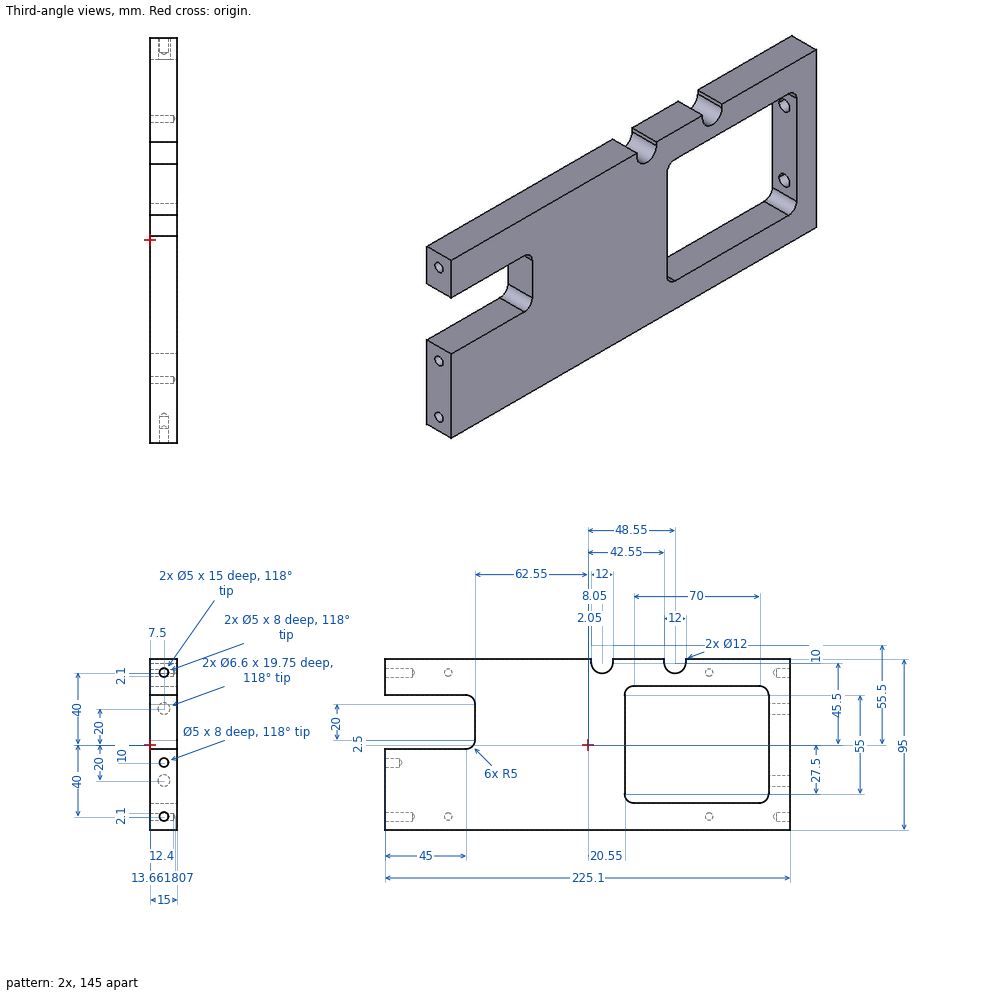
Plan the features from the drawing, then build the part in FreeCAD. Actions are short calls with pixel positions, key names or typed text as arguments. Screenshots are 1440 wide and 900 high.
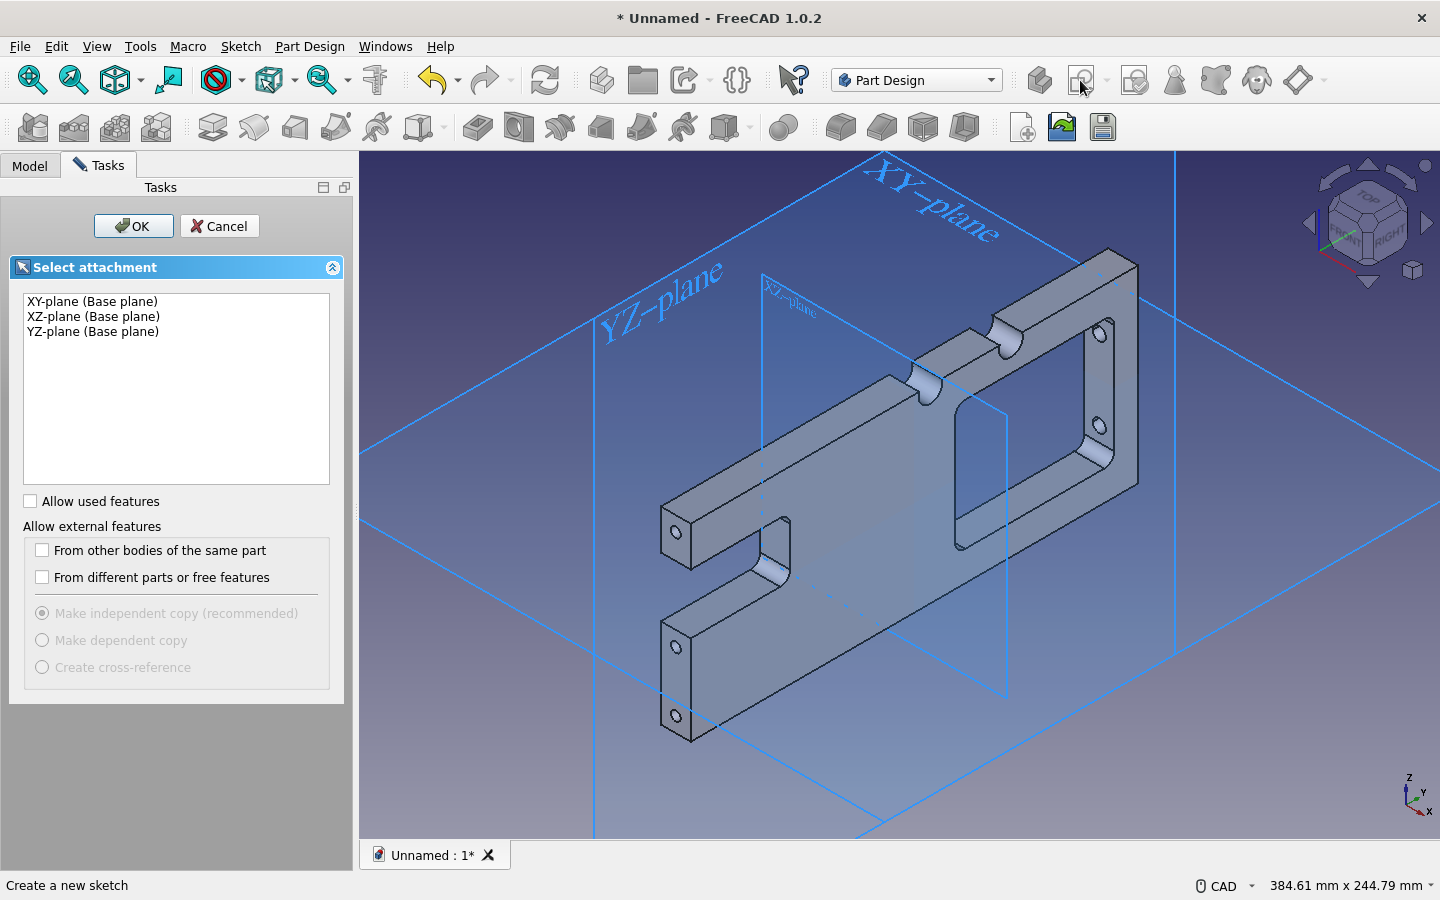
click(84, 332)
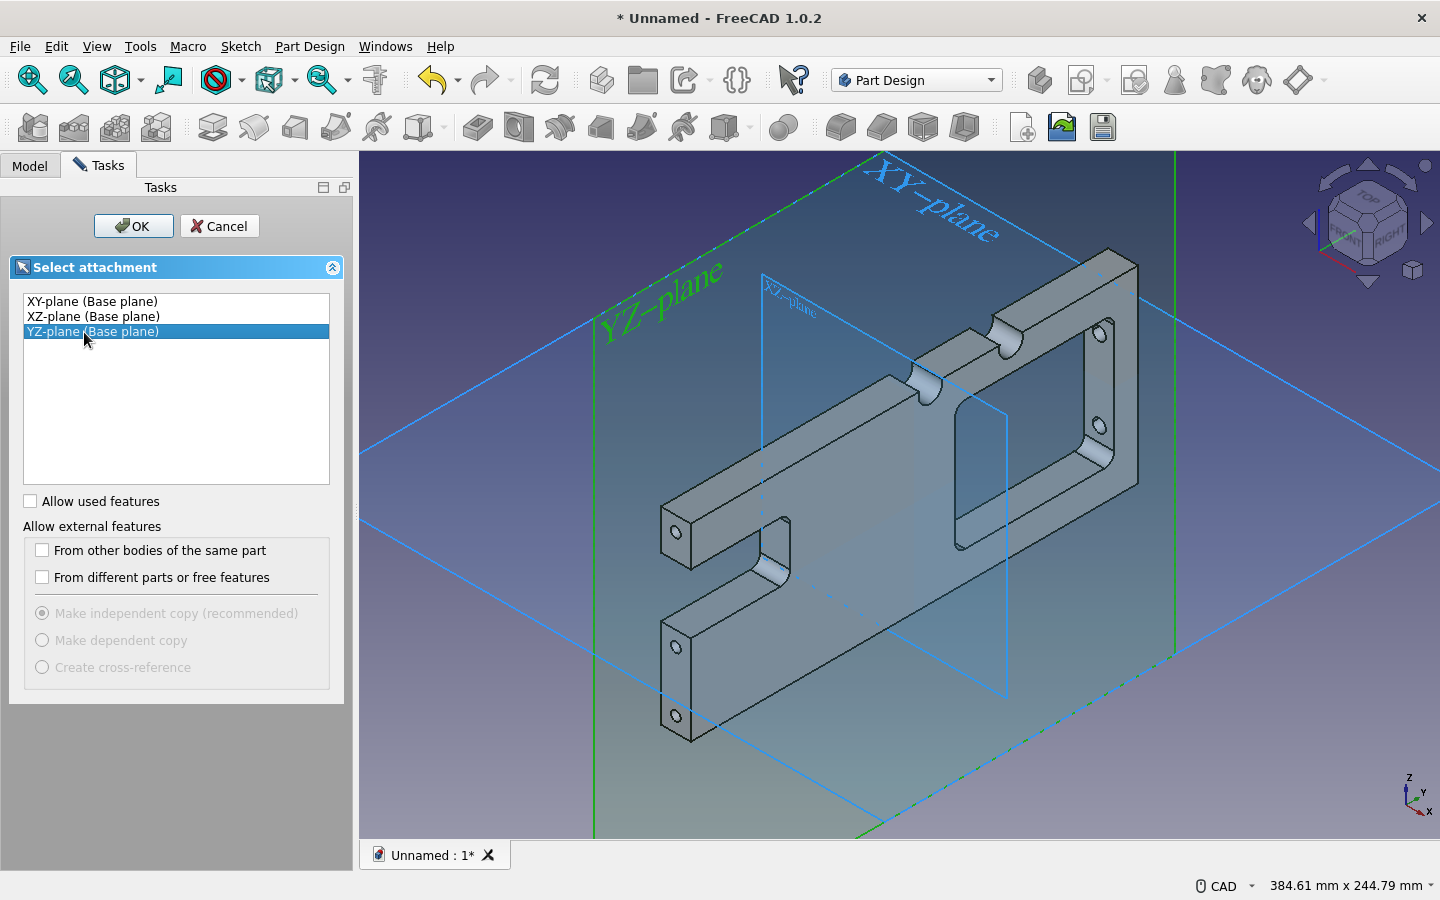
click(134, 226)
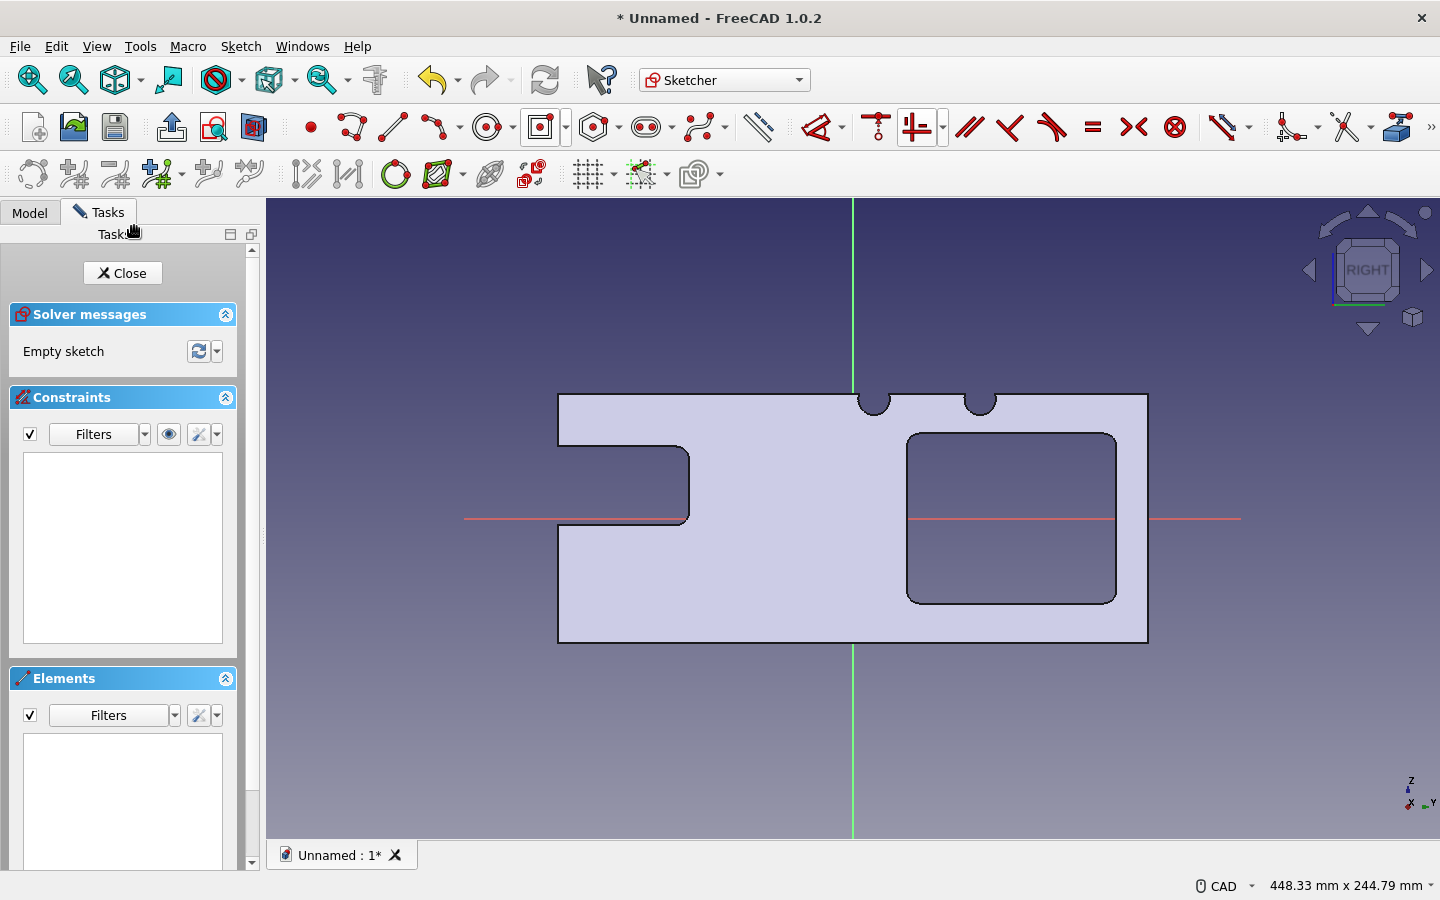
click(254, 128)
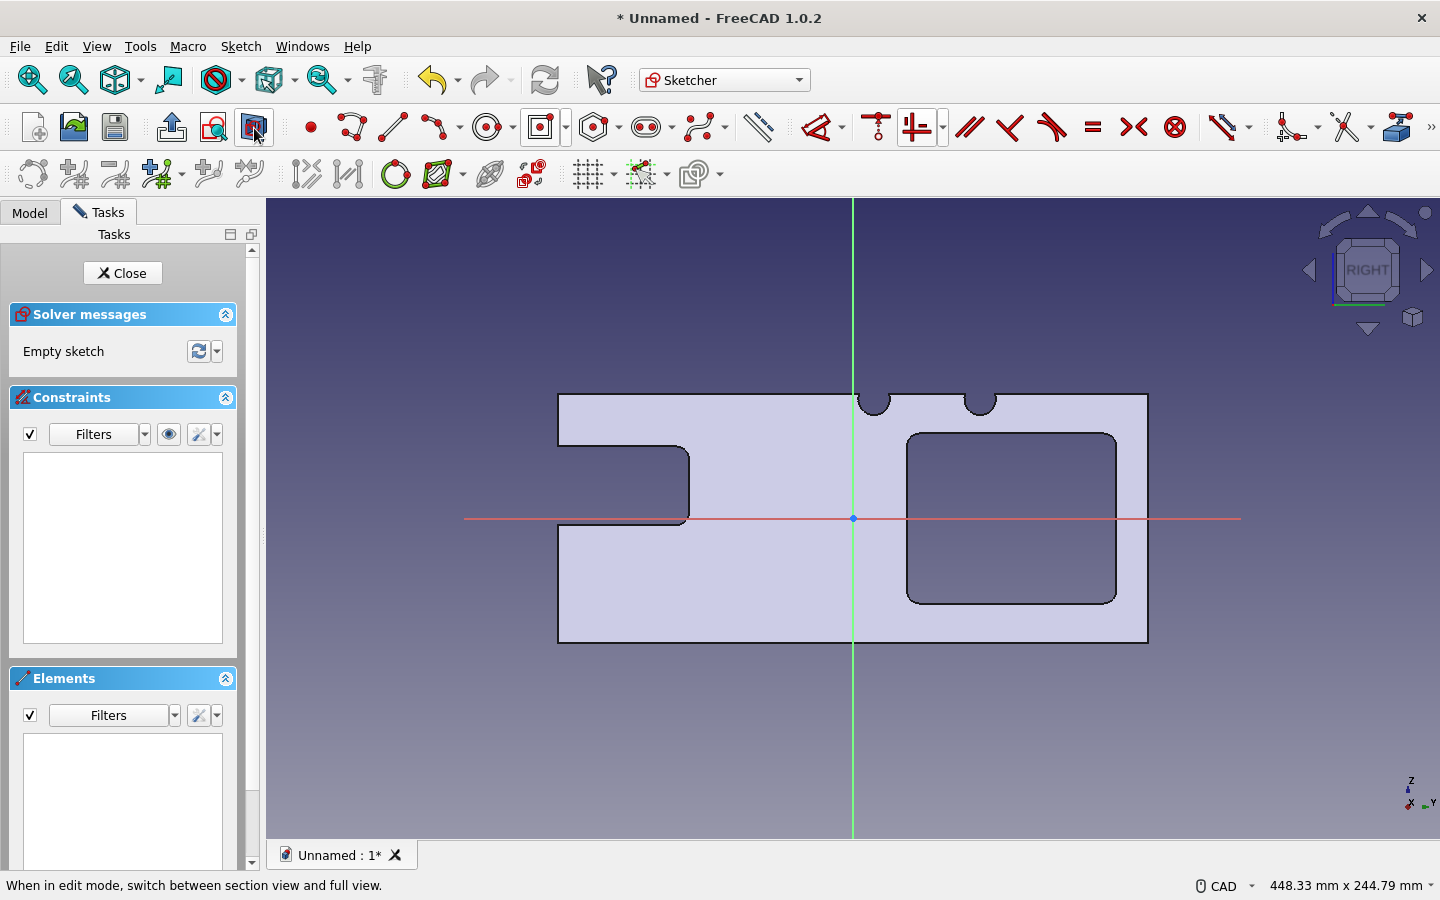
scroll(1006, 404, up, 5)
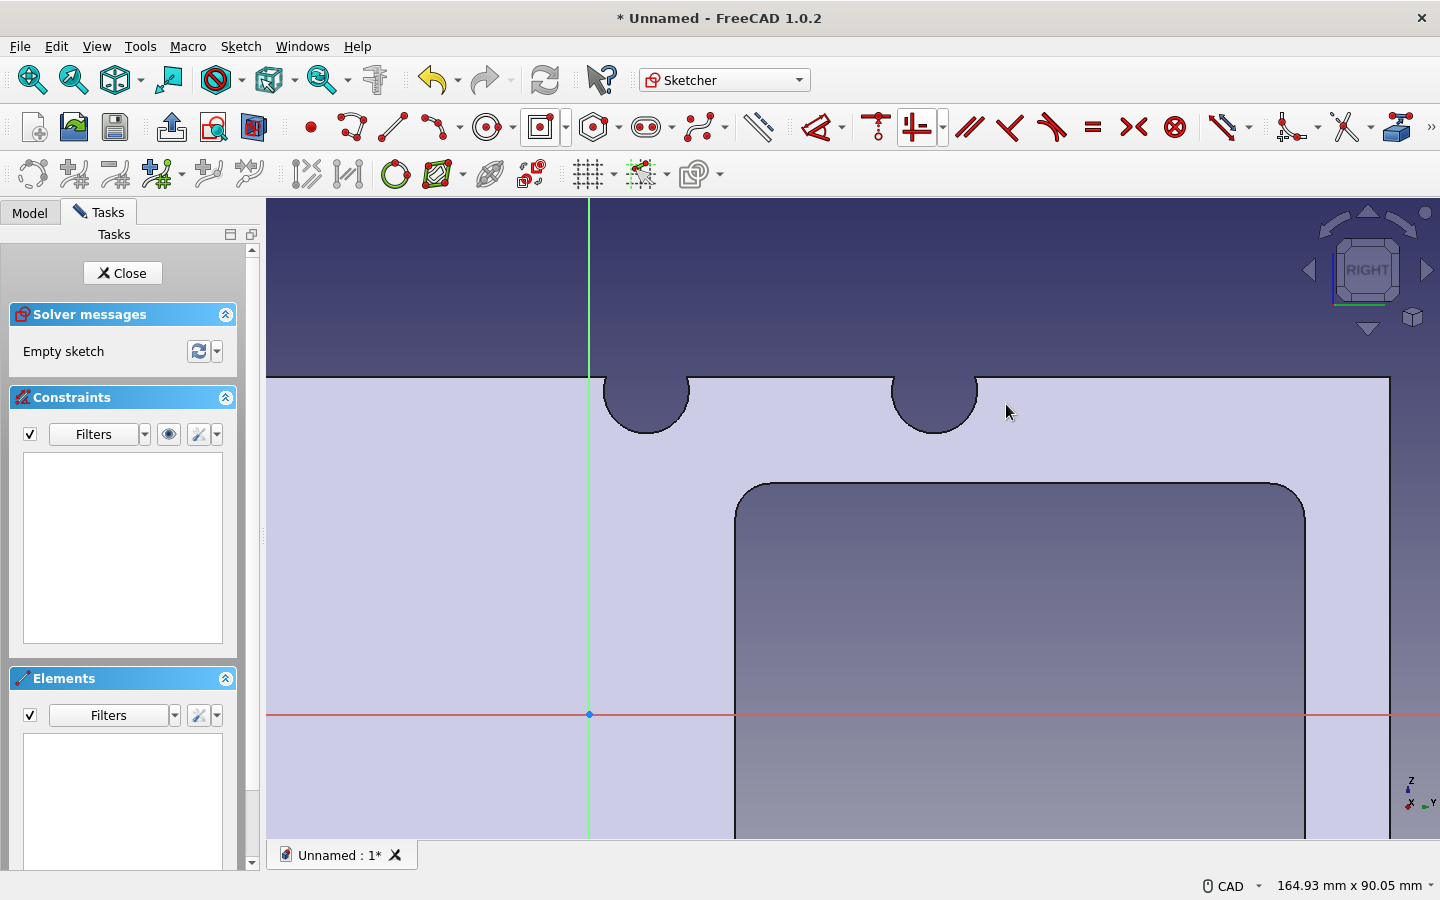
click(566, 128)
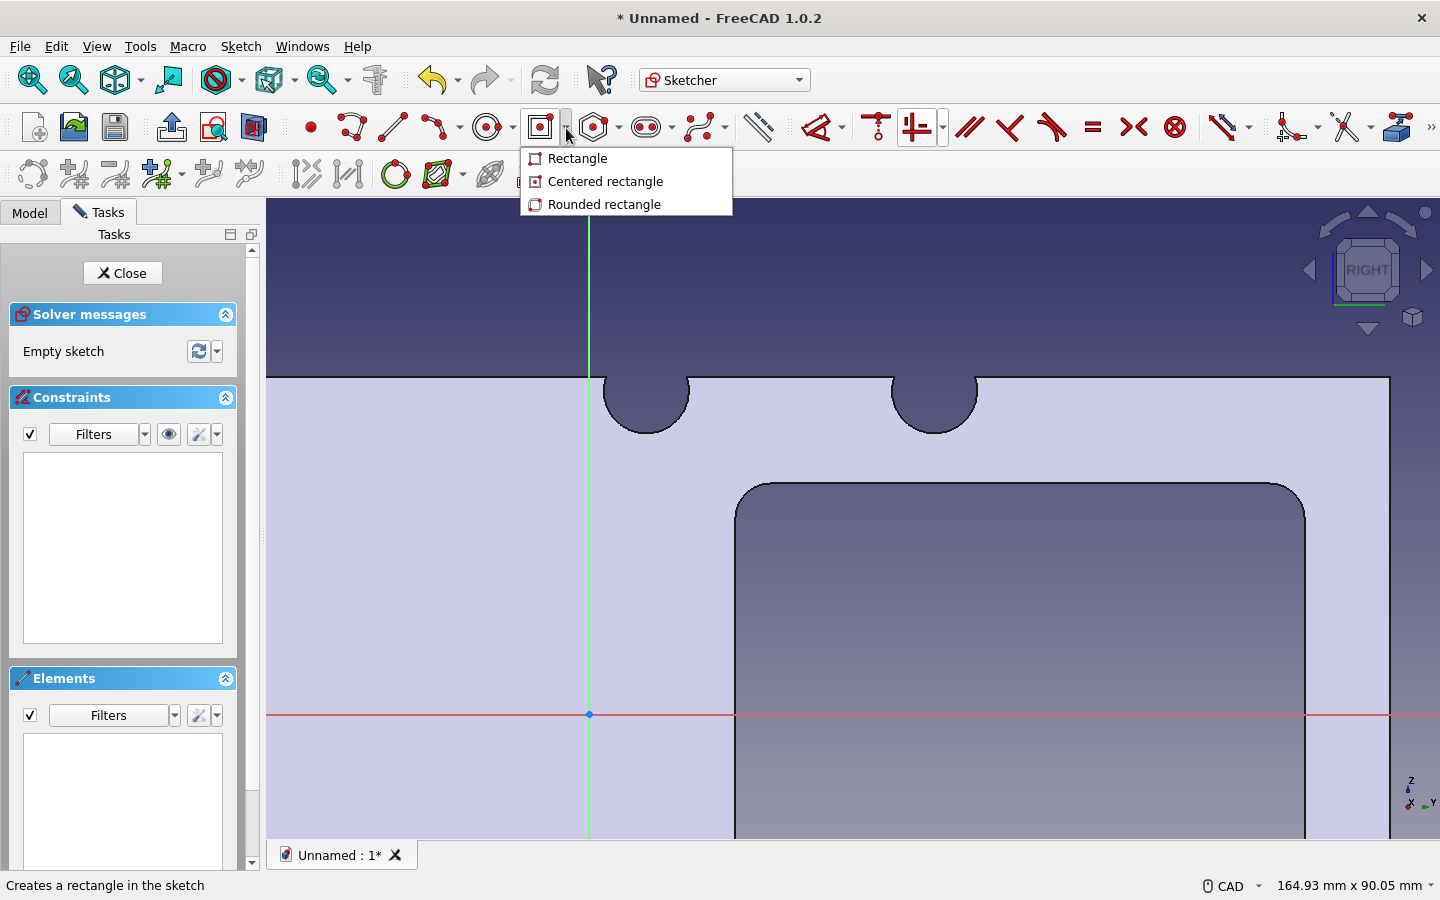
click(626, 158)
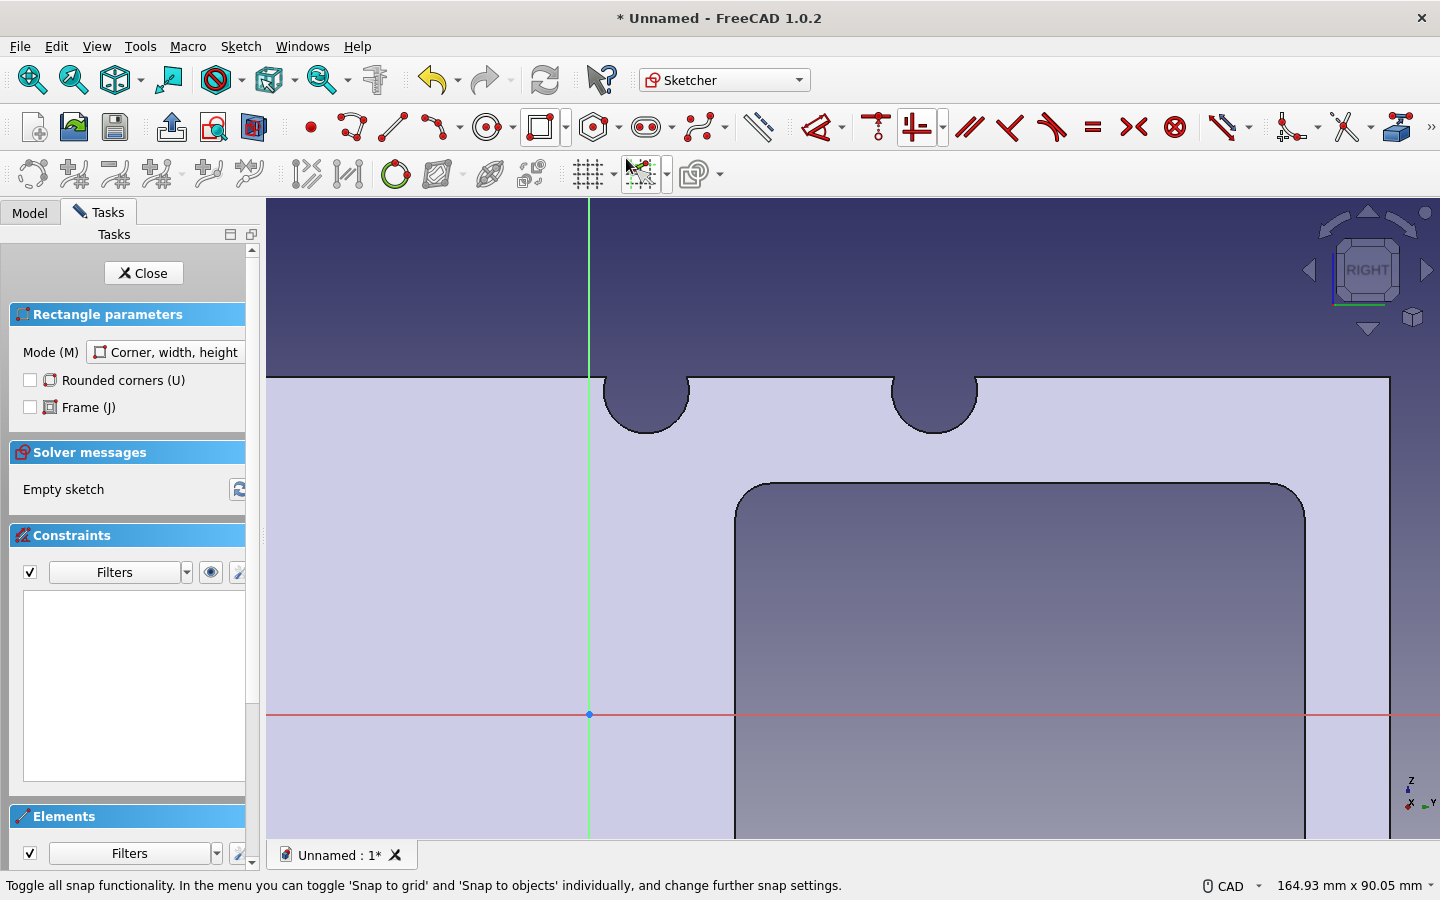
click(604, 320)
move(689, 391)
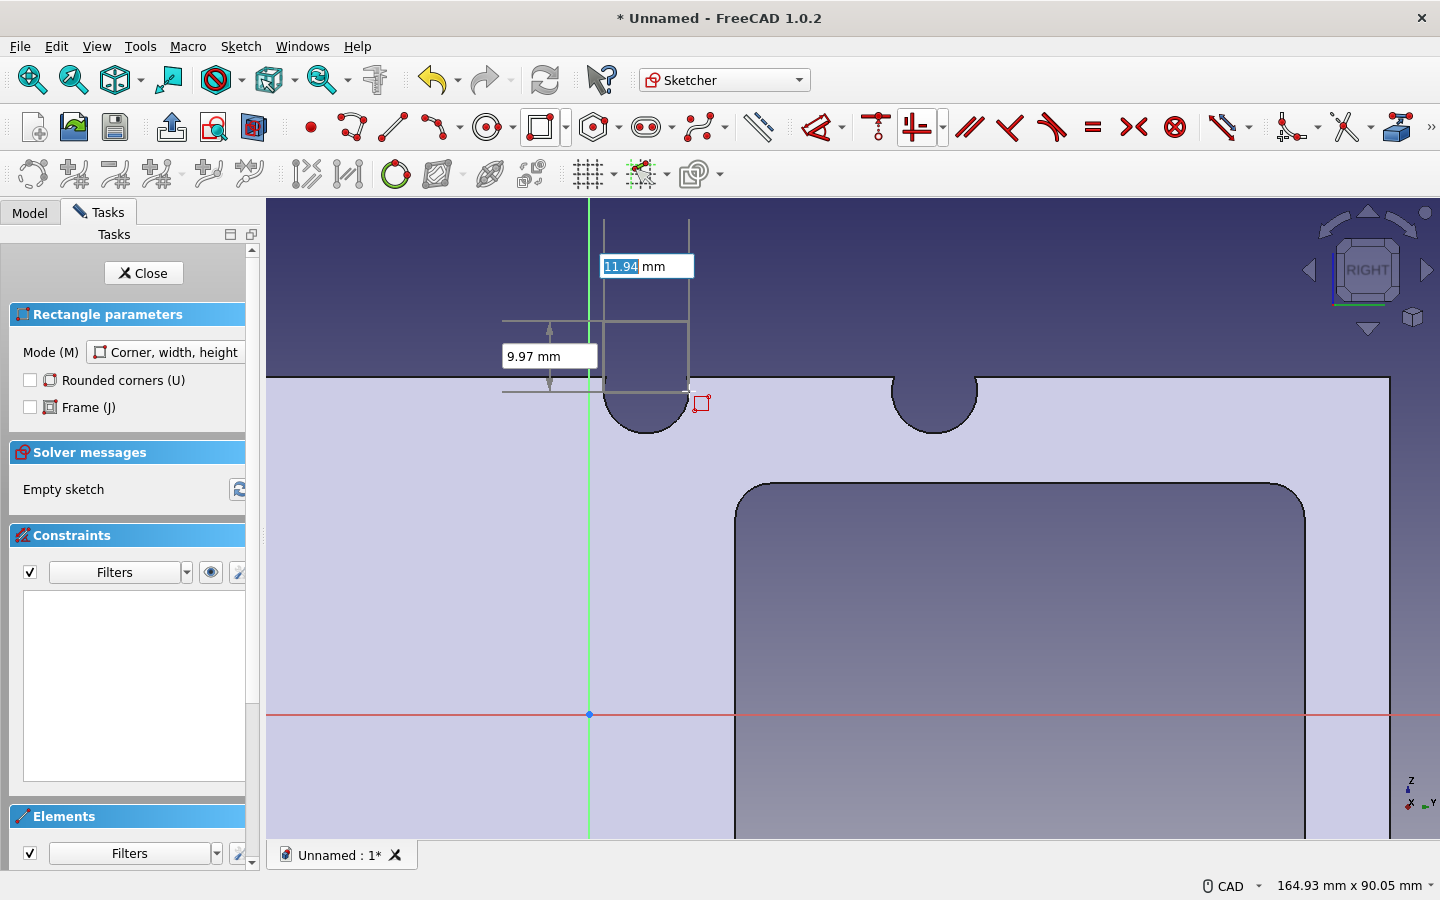
text(12)
key(Tab)
text(10)
key(Return)